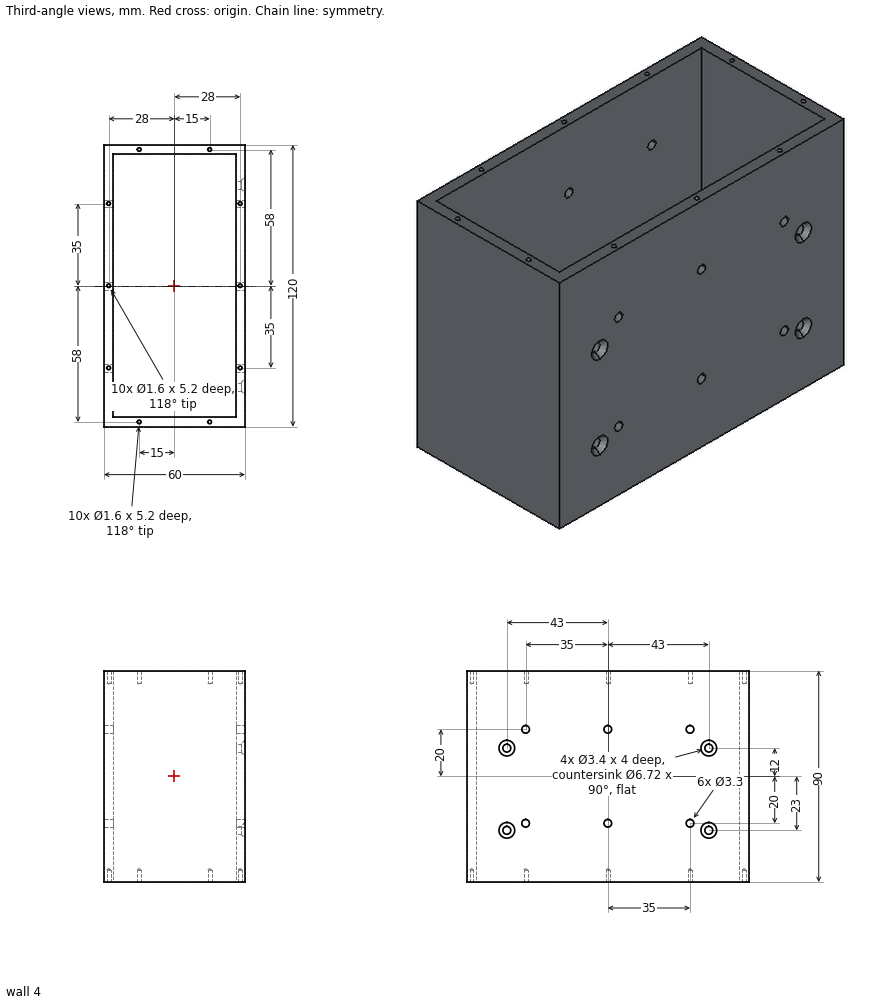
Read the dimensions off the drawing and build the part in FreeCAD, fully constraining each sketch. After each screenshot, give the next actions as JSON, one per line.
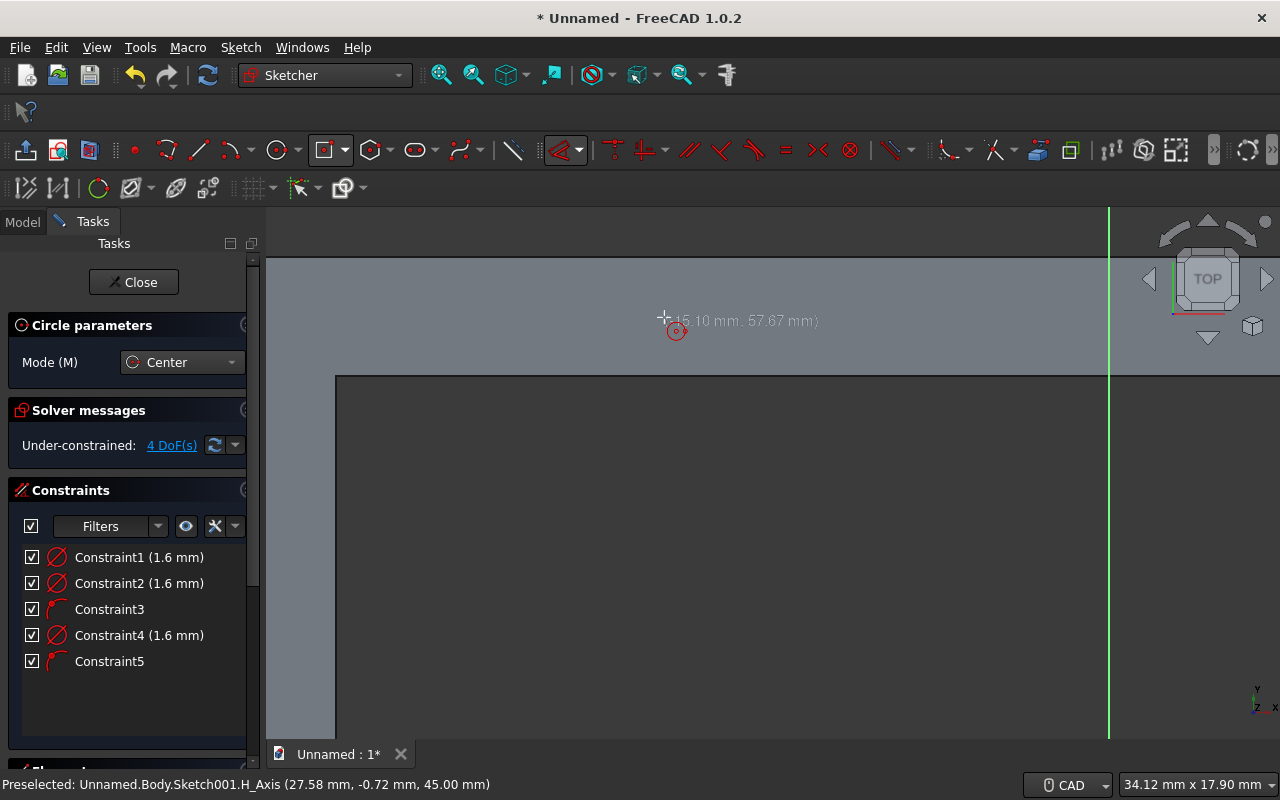
{"action": "scroll", "coordinate": [664, 317], "scroll_direction": "down", "scroll_amount": 12}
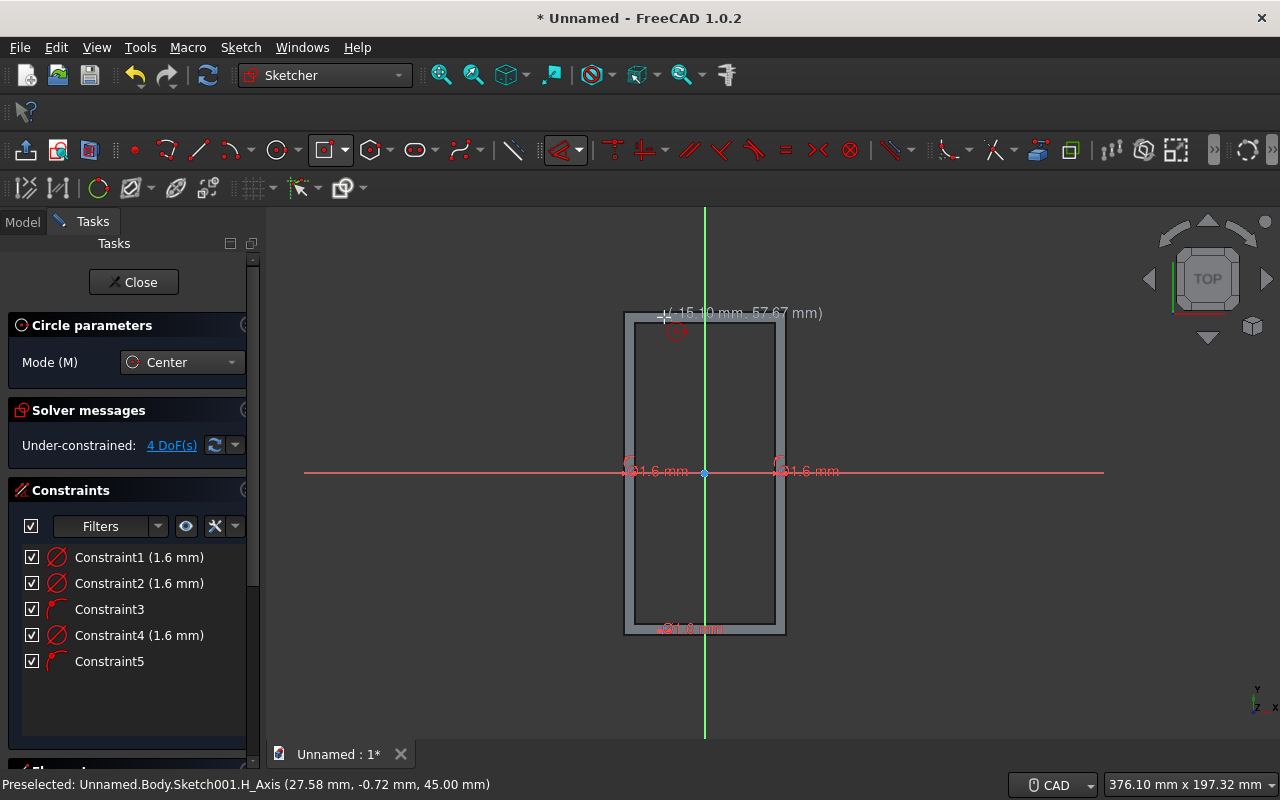
{"action": "left_click", "coordinate": [664, 317]}
{"action": "mouse_move", "coordinate": [666, 316]}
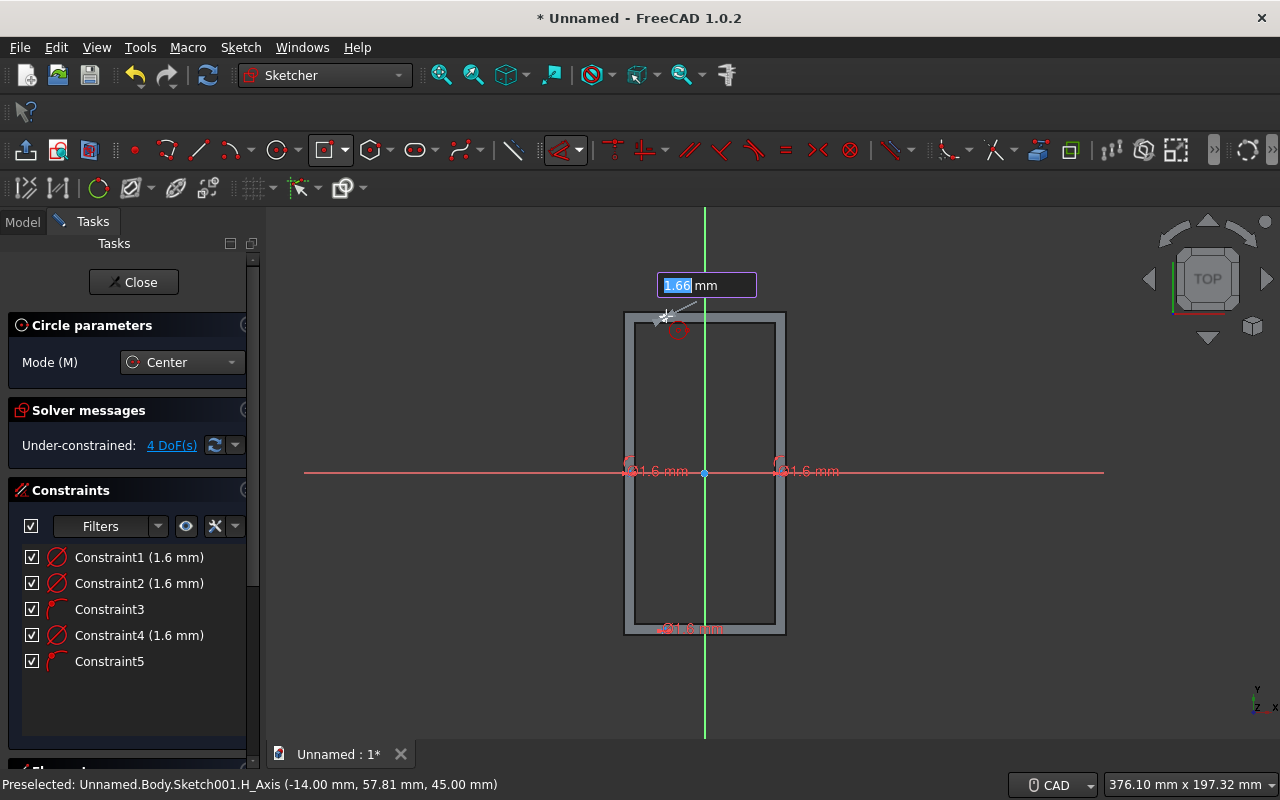
{"action": "type", "text": "1.6"}
{"action": "key", "text": "Return"}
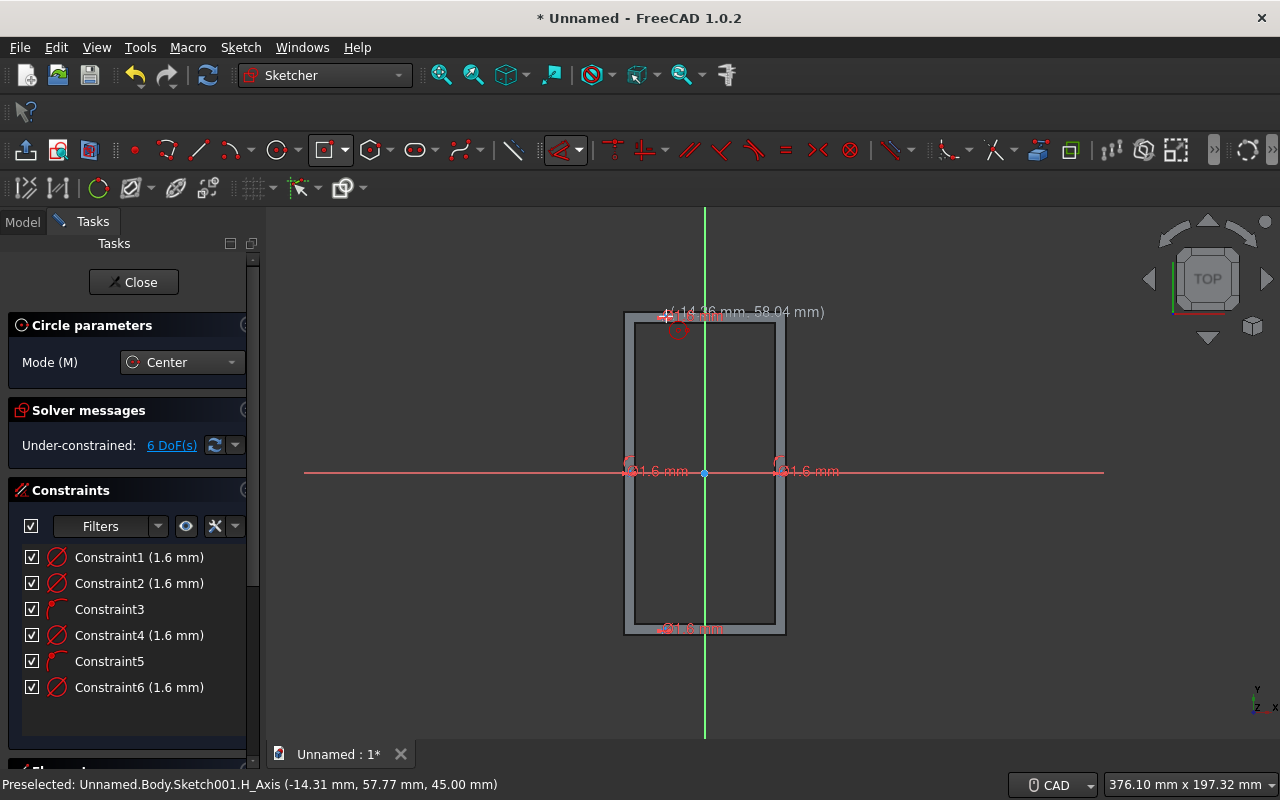
{"action": "scroll", "coordinate": [745, 317], "scroll_direction": "up", "scroll_amount": 12}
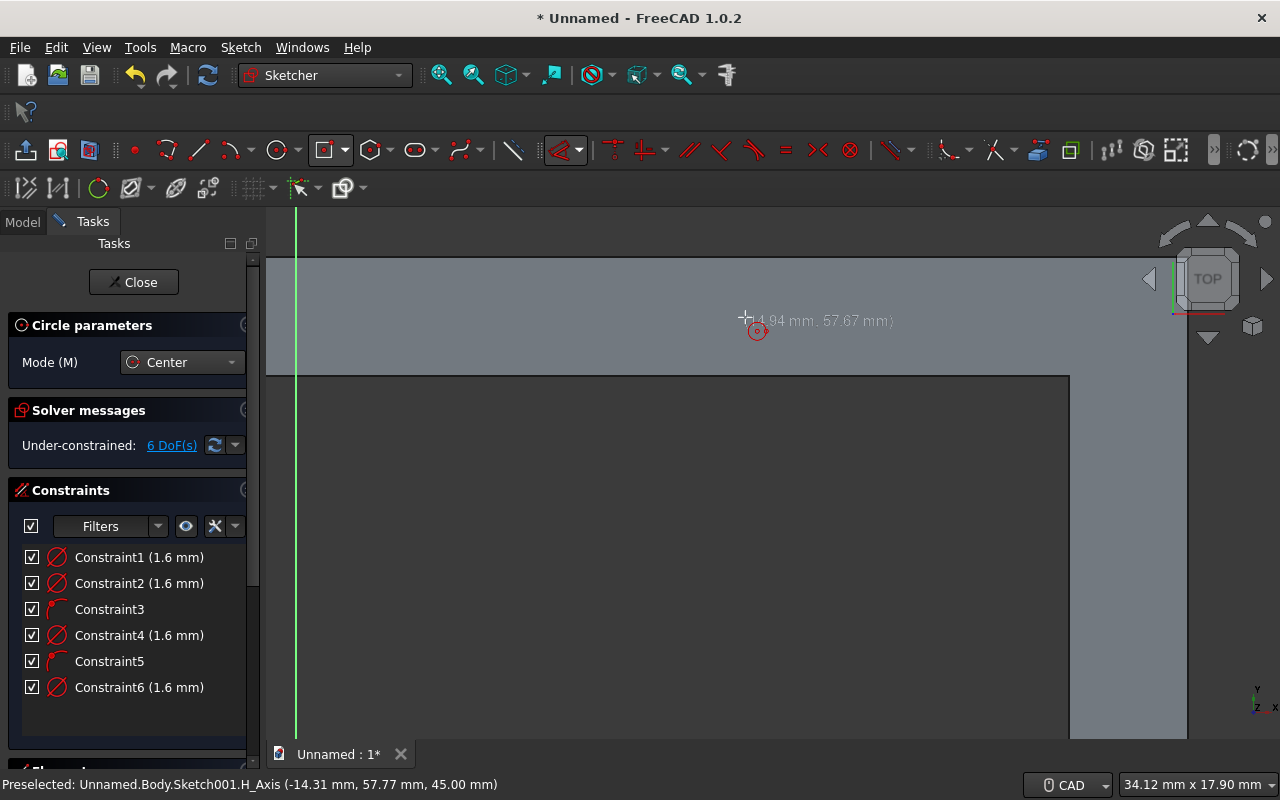
{"action": "scroll", "coordinate": [745, 317], "scroll_direction": "down", "scroll_amount": 12}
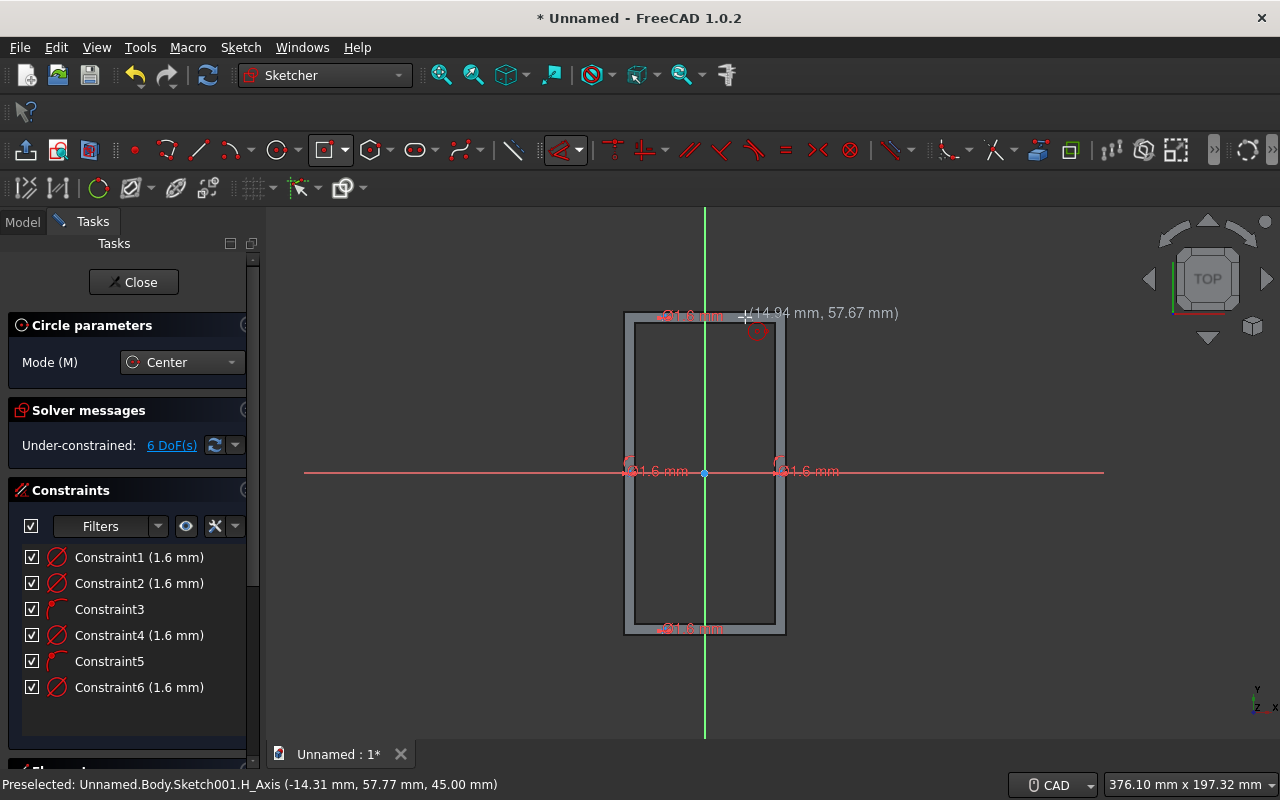
{"action": "left_click", "coordinate": [745, 317]}
{"action": "mouse_move", "coordinate": [747, 316]}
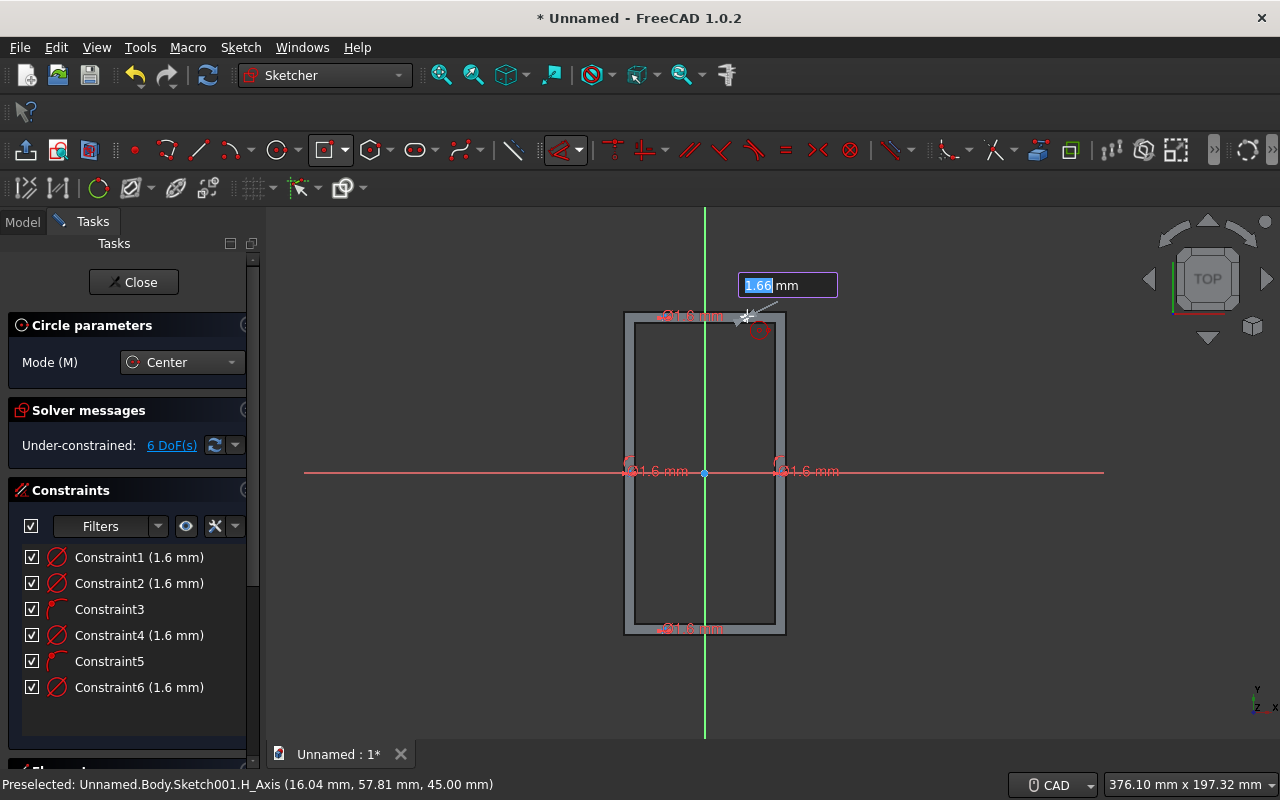
{"action": "type", "text": "1.6"}
{"action": "key", "text": "Return"}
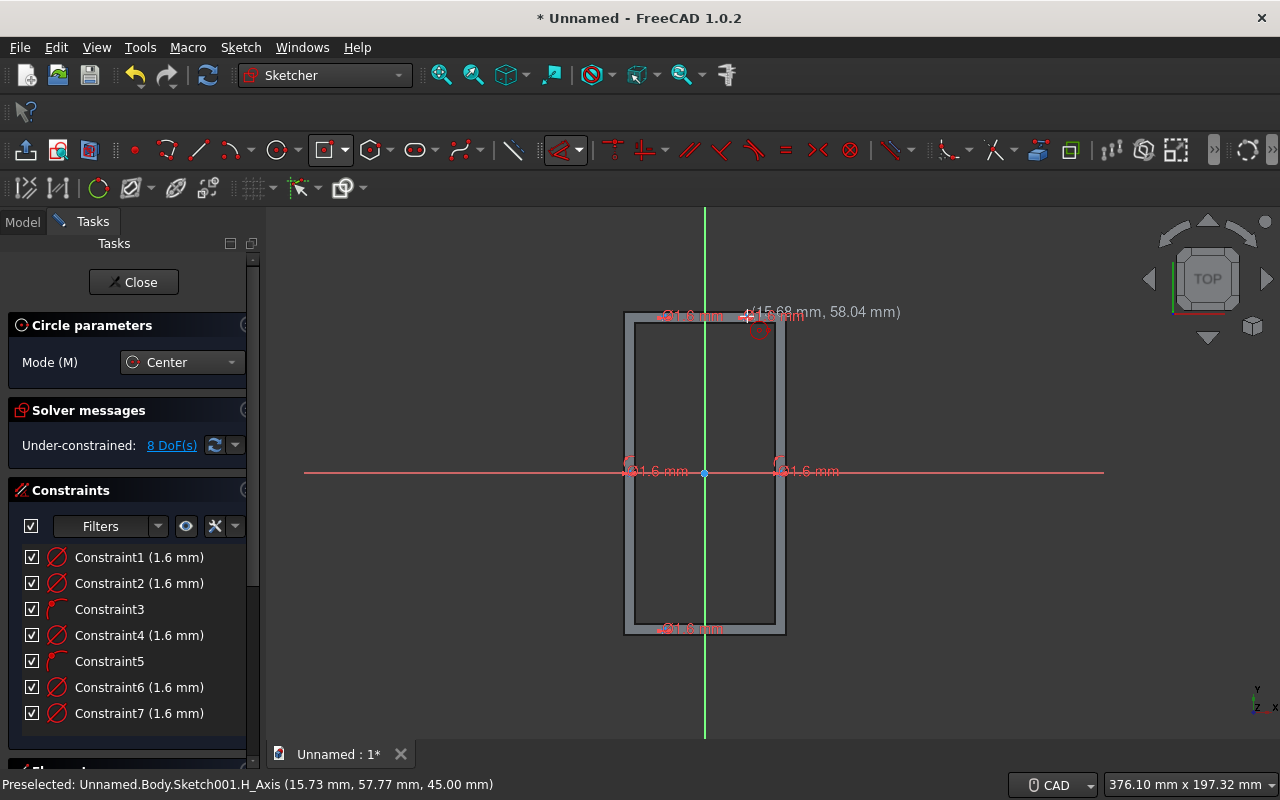
{"action": "scroll", "coordinate": [629, 379], "scroll_direction": "up", "scroll_amount": 12}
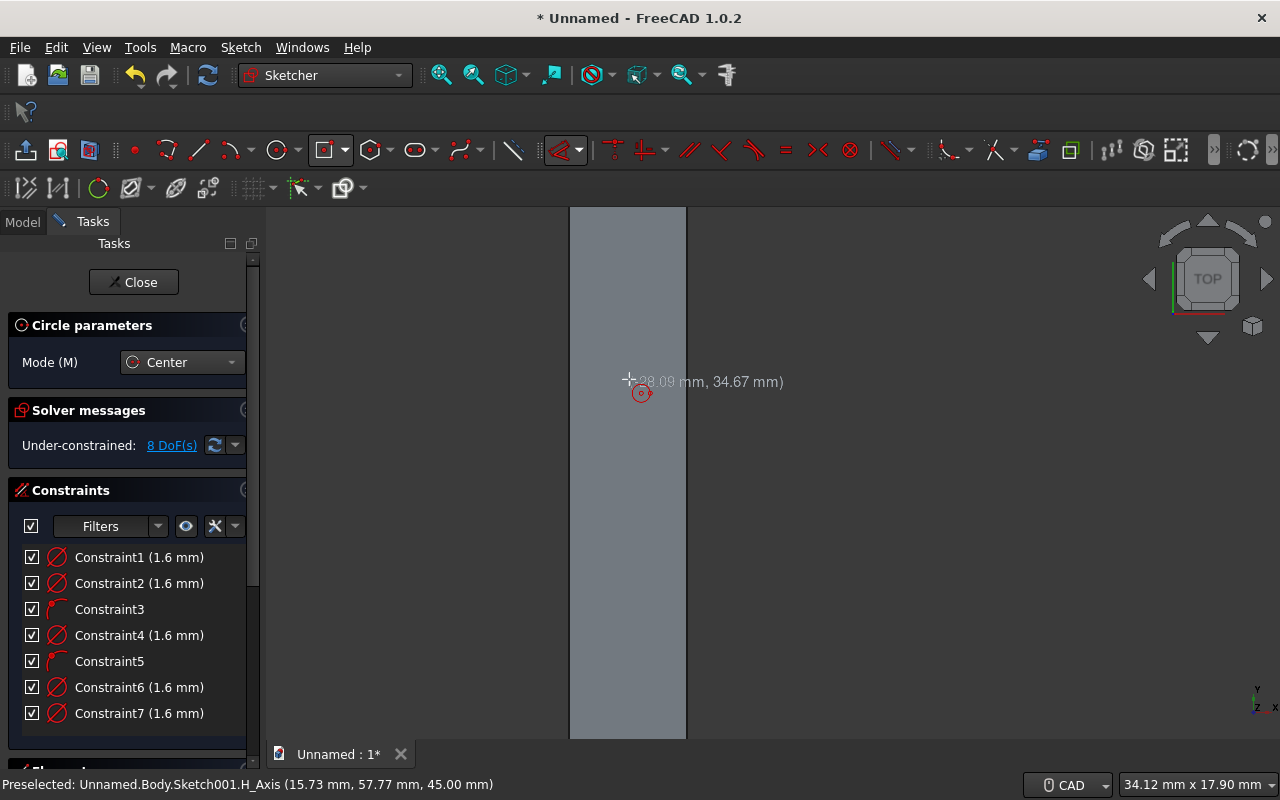
{"action": "scroll", "coordinate": [629, 379], "scroll_direction": "down", "scroll_amount": 12}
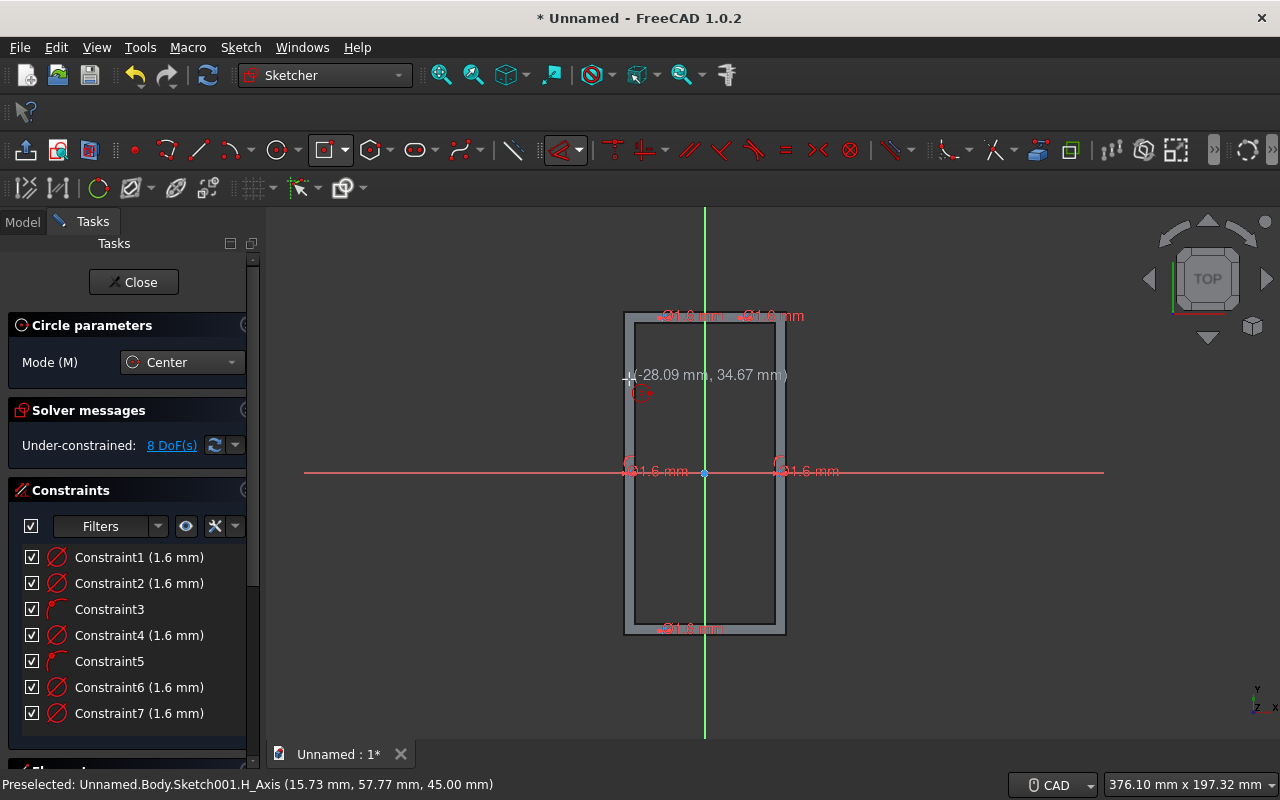
{"action": "left_click", "coordinate": [629, 379]}
{"action": "mouse_move", "coordinate": [631, 378]}